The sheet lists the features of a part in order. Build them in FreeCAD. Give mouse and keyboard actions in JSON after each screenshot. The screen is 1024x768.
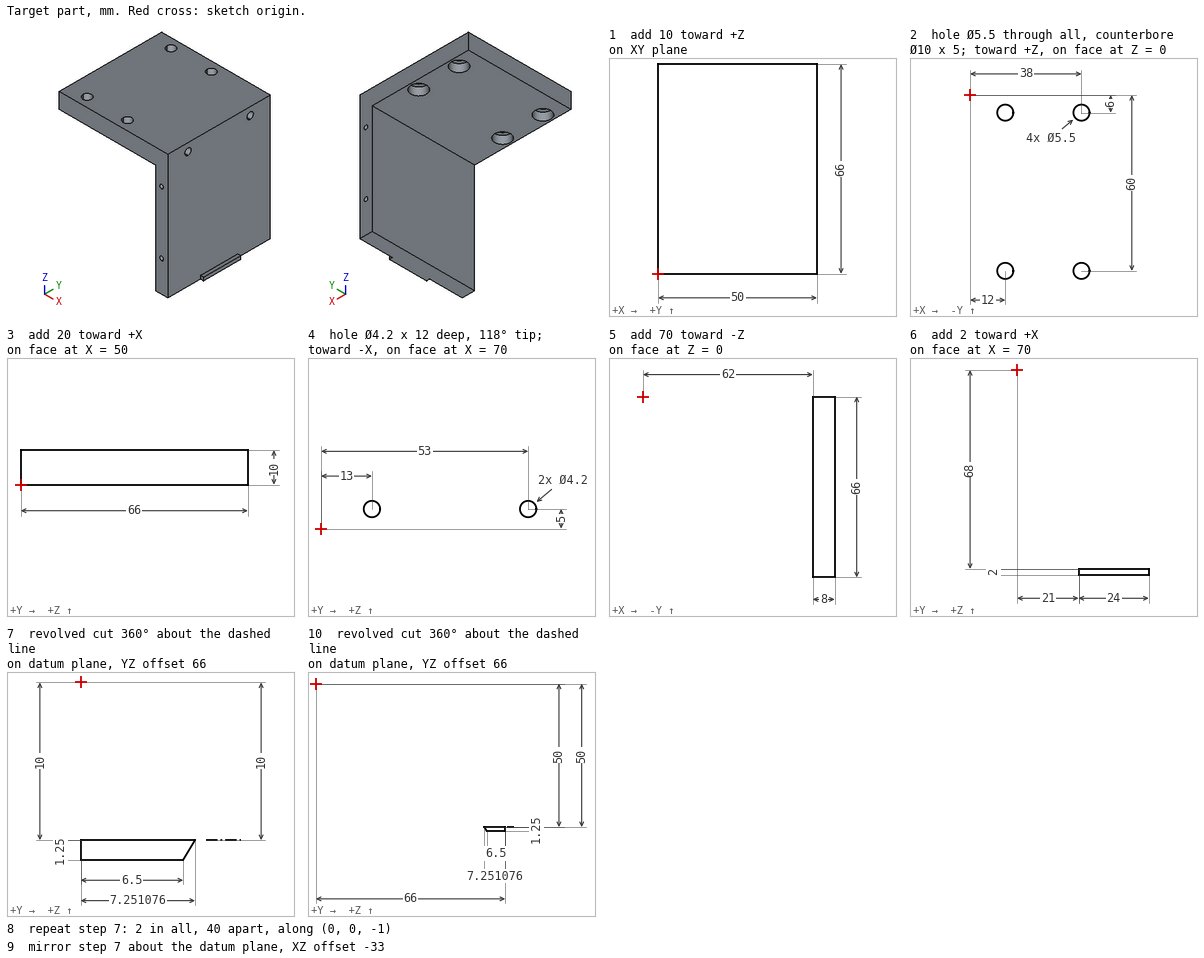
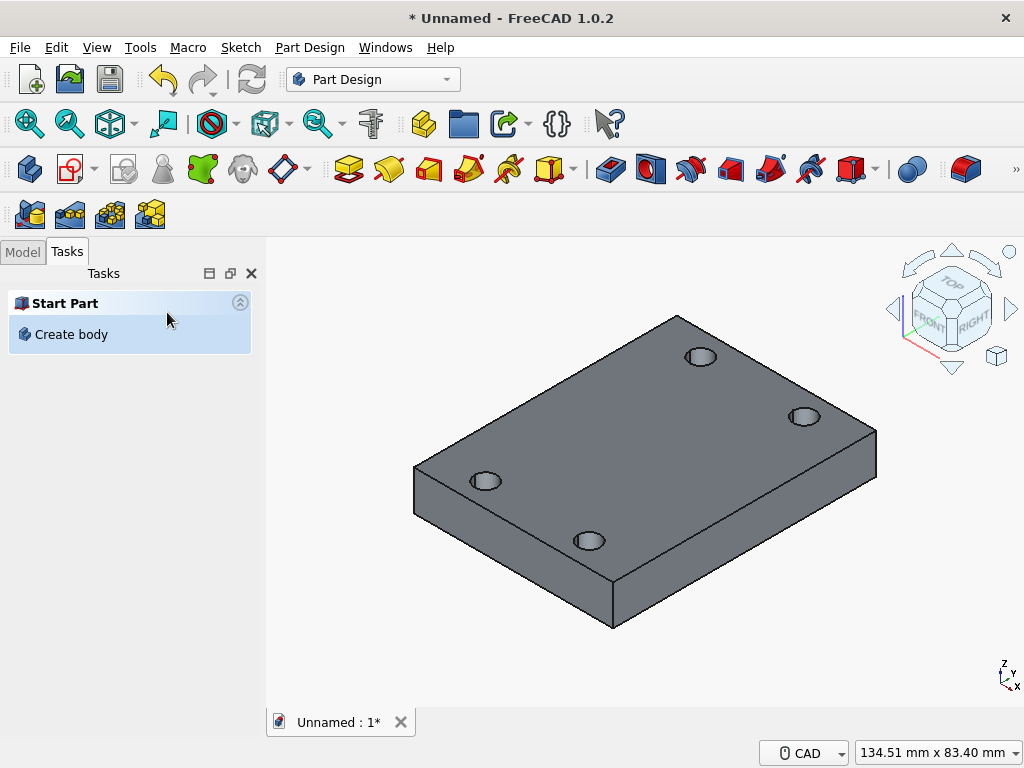
{"action": "left_click", "coordinate": [820, 485]}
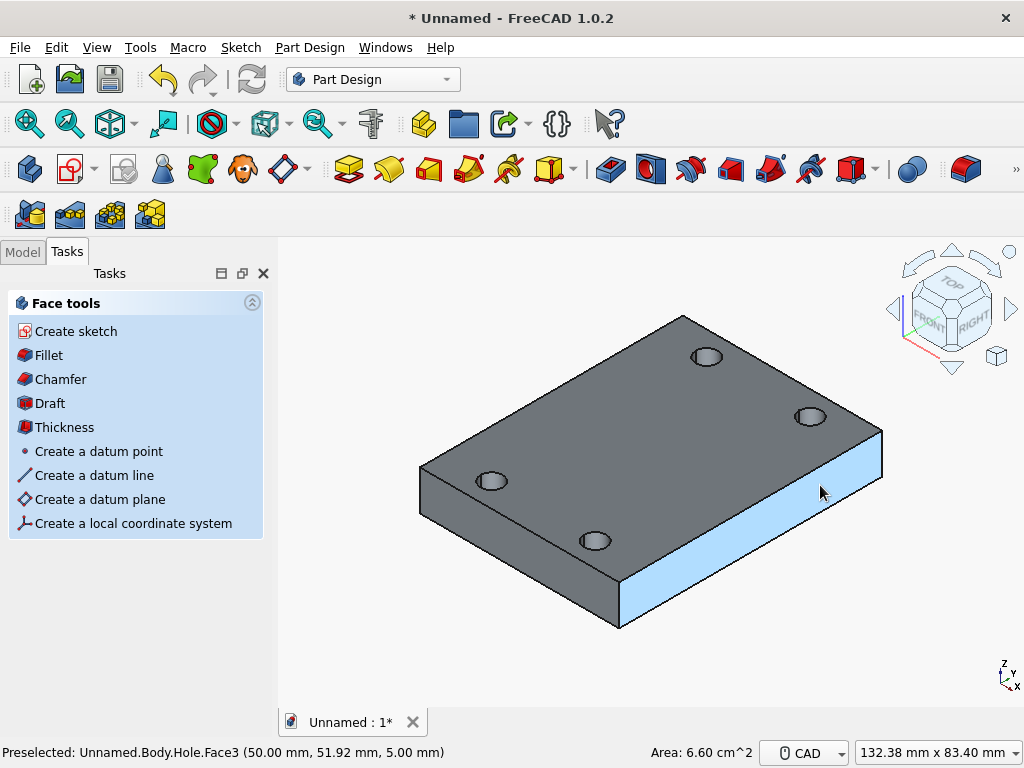
{"action": "left_click", "coordinate": [70, 170]}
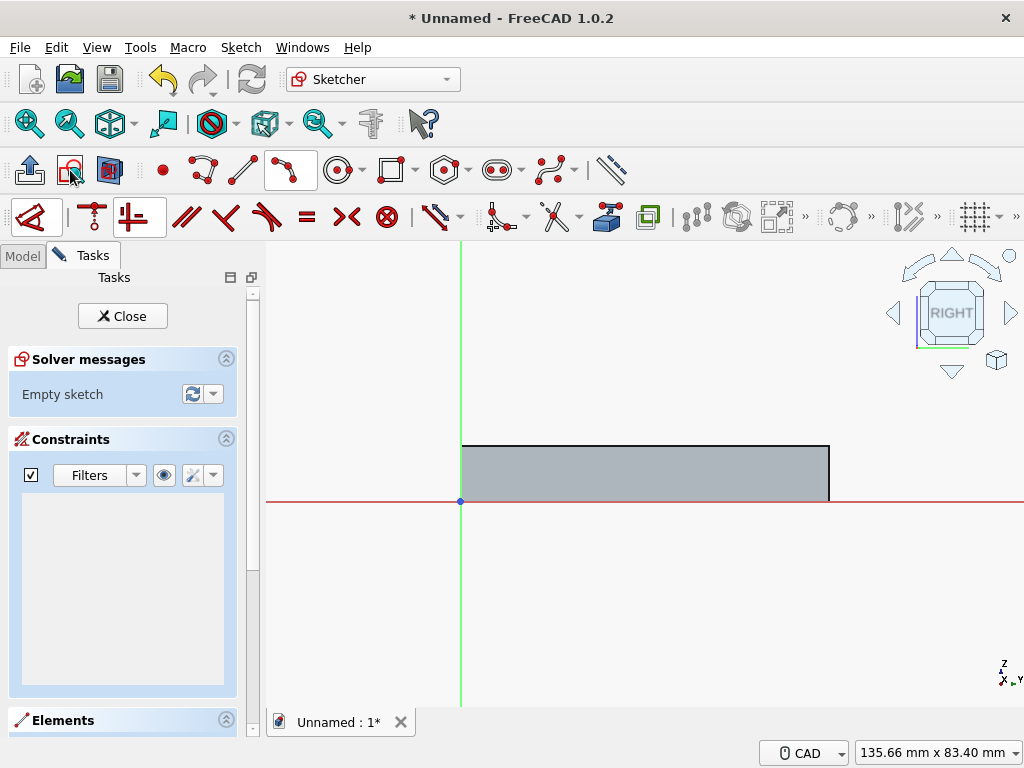
{"action": "left_click", "coordinate": [392, 170]}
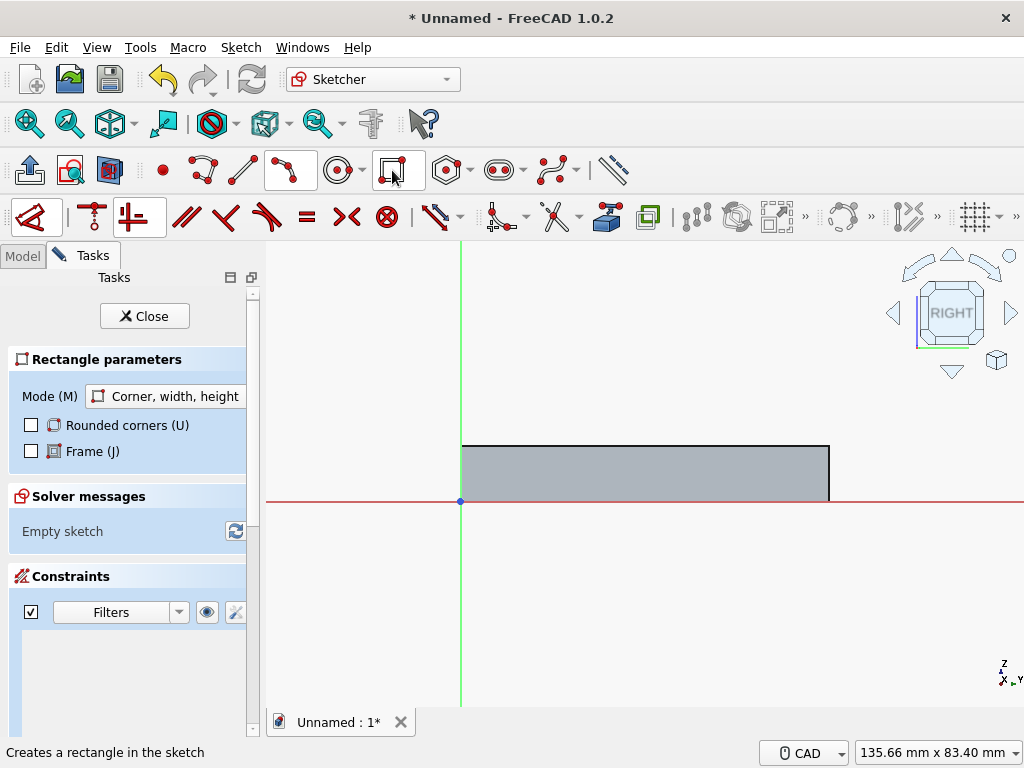
{"action": "left_click", "coordinate": [461, 502]}
{"action": "left_click", "coordinate": [829, 446]}
{"action": "key", "text": "Escape"}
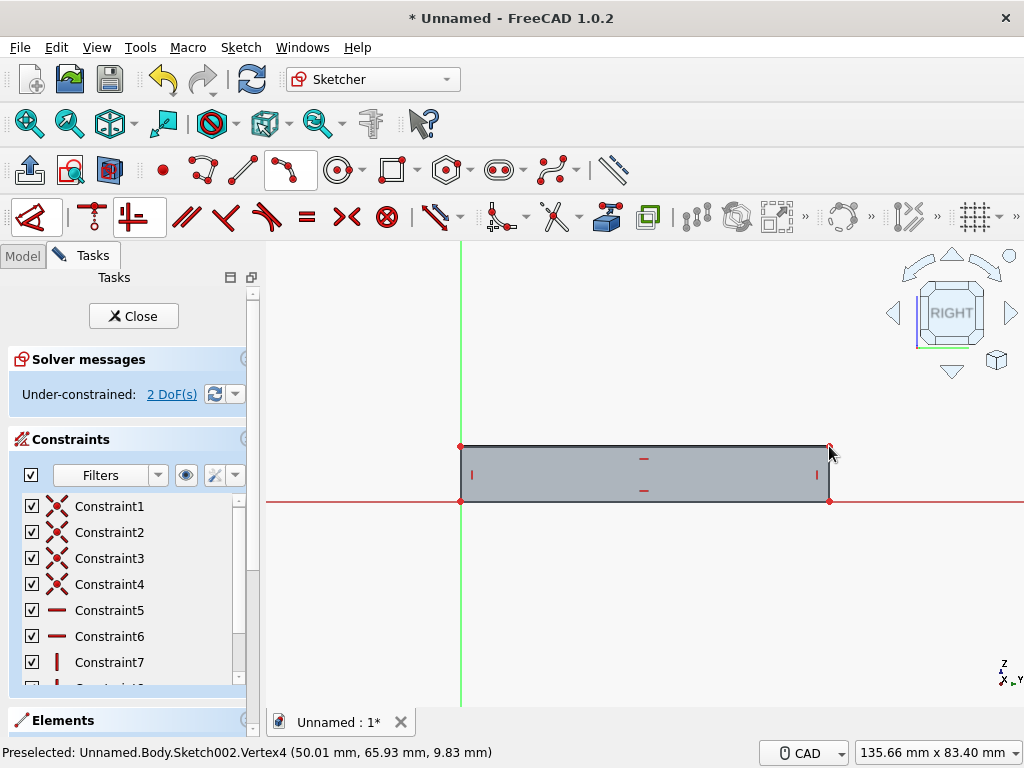
{"action": "left_click", "coordinate": [571, 502]}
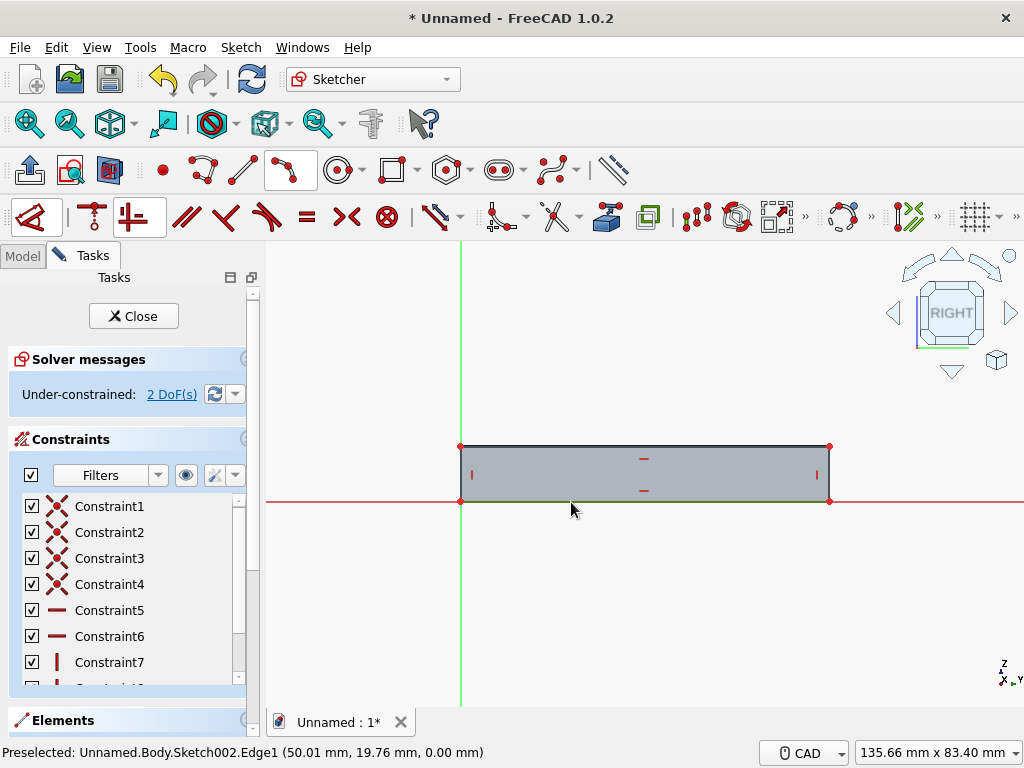
{"action": "key", "text": "l"}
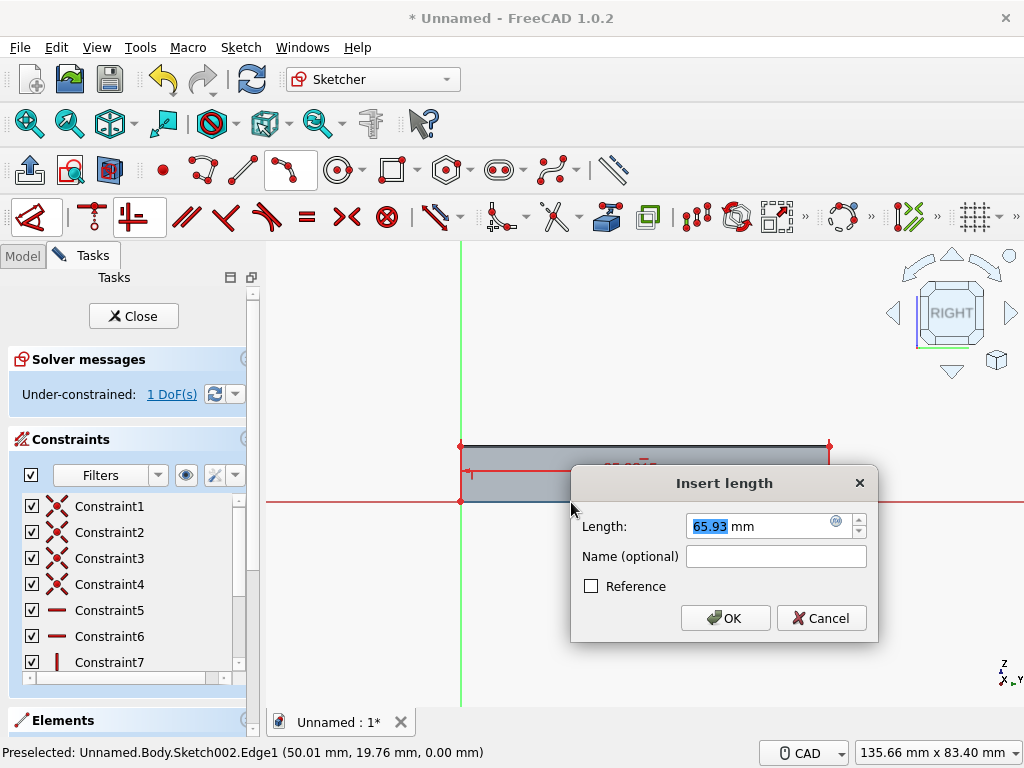
{"action": "type", "text": "66"}
{"action": "key", "text": "Return"}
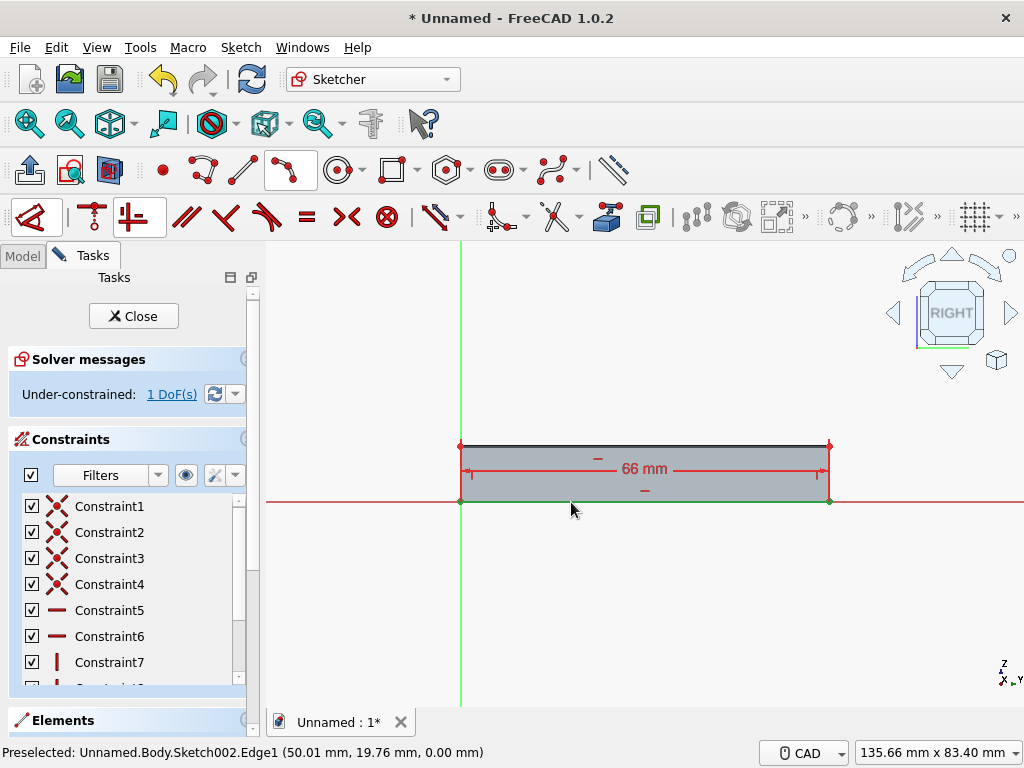
{"action": "left_click", "coordinate": [829, 485]}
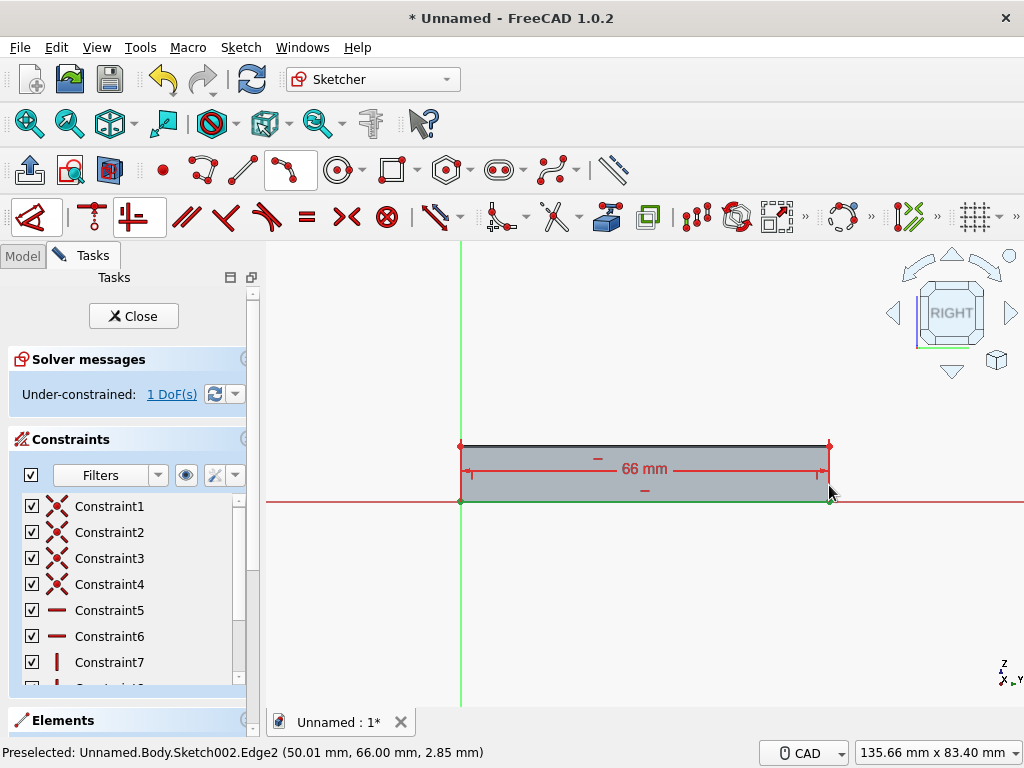
{"action": "key", "text": "i"}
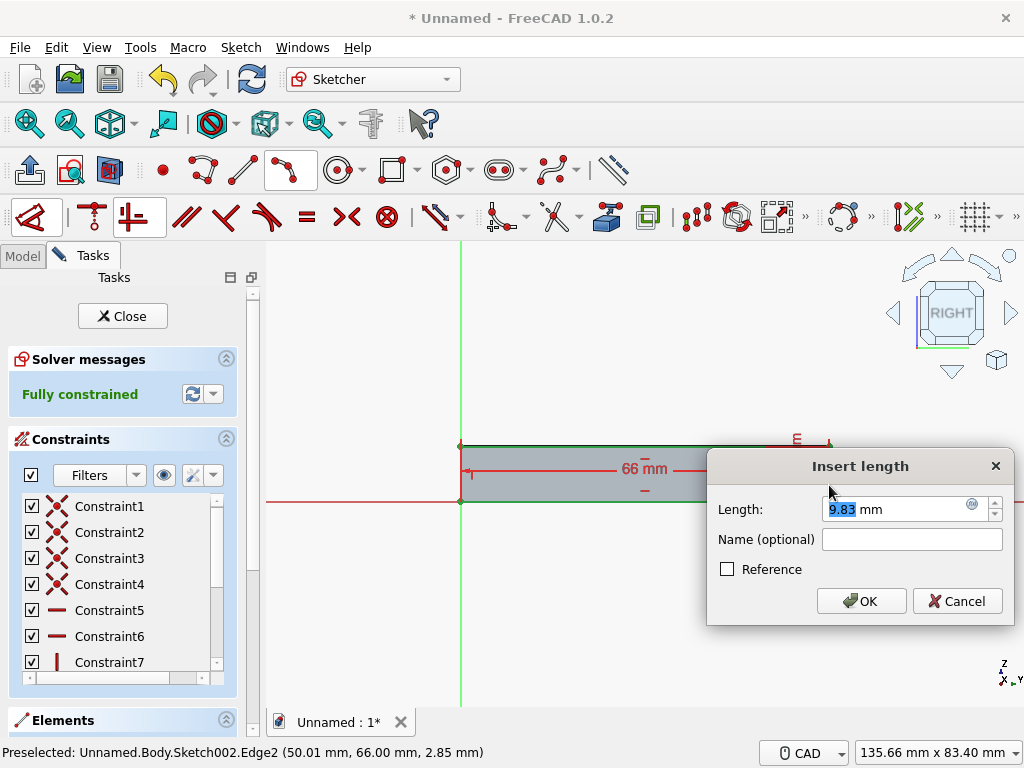
{"action": "type", "text": "10"}
{"action": "key", "text": "Return"}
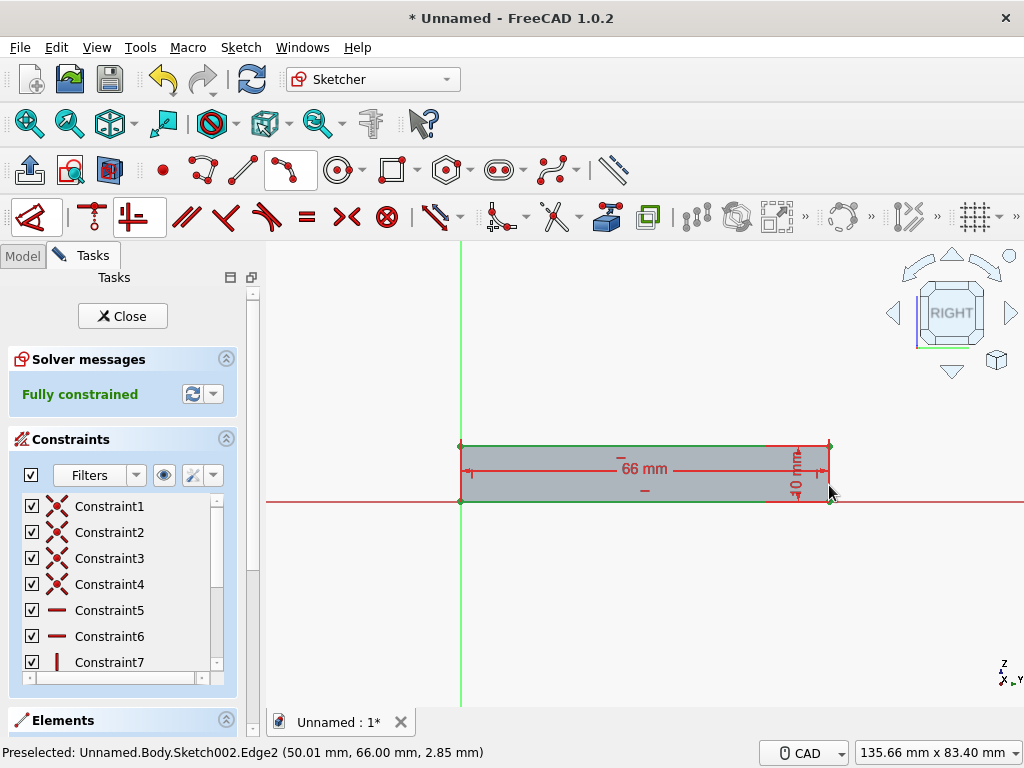
{"action": "left_click", "coordinate": [123, 316]}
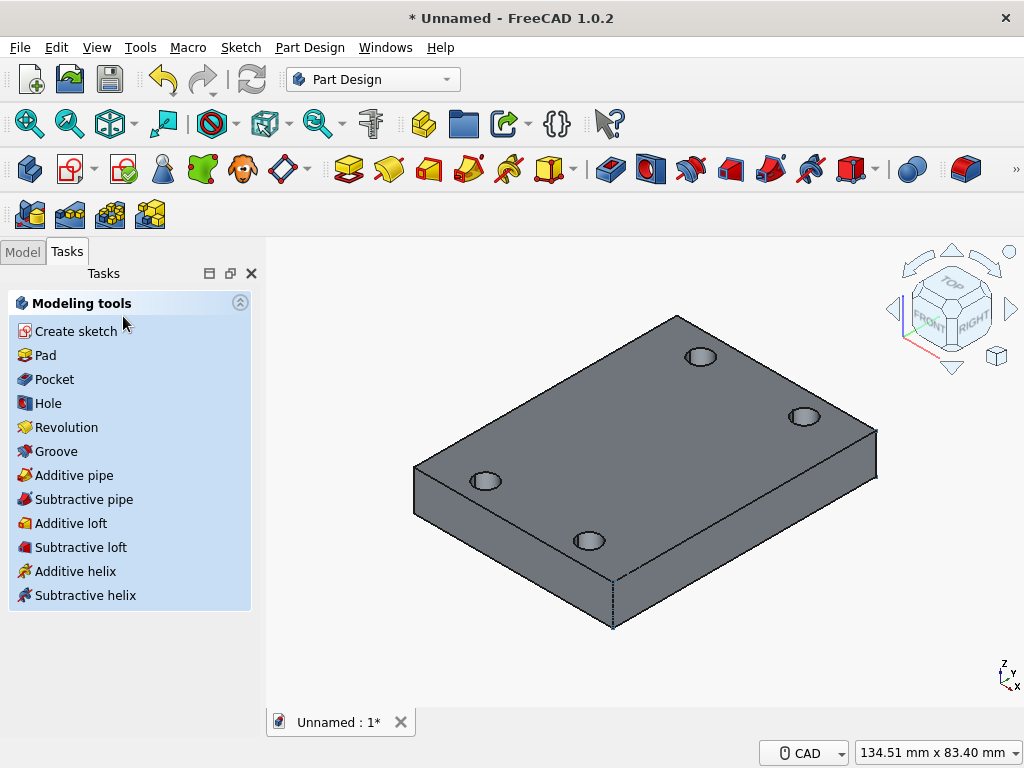
{"action": "left_click", "coordinate": [350, 170]}